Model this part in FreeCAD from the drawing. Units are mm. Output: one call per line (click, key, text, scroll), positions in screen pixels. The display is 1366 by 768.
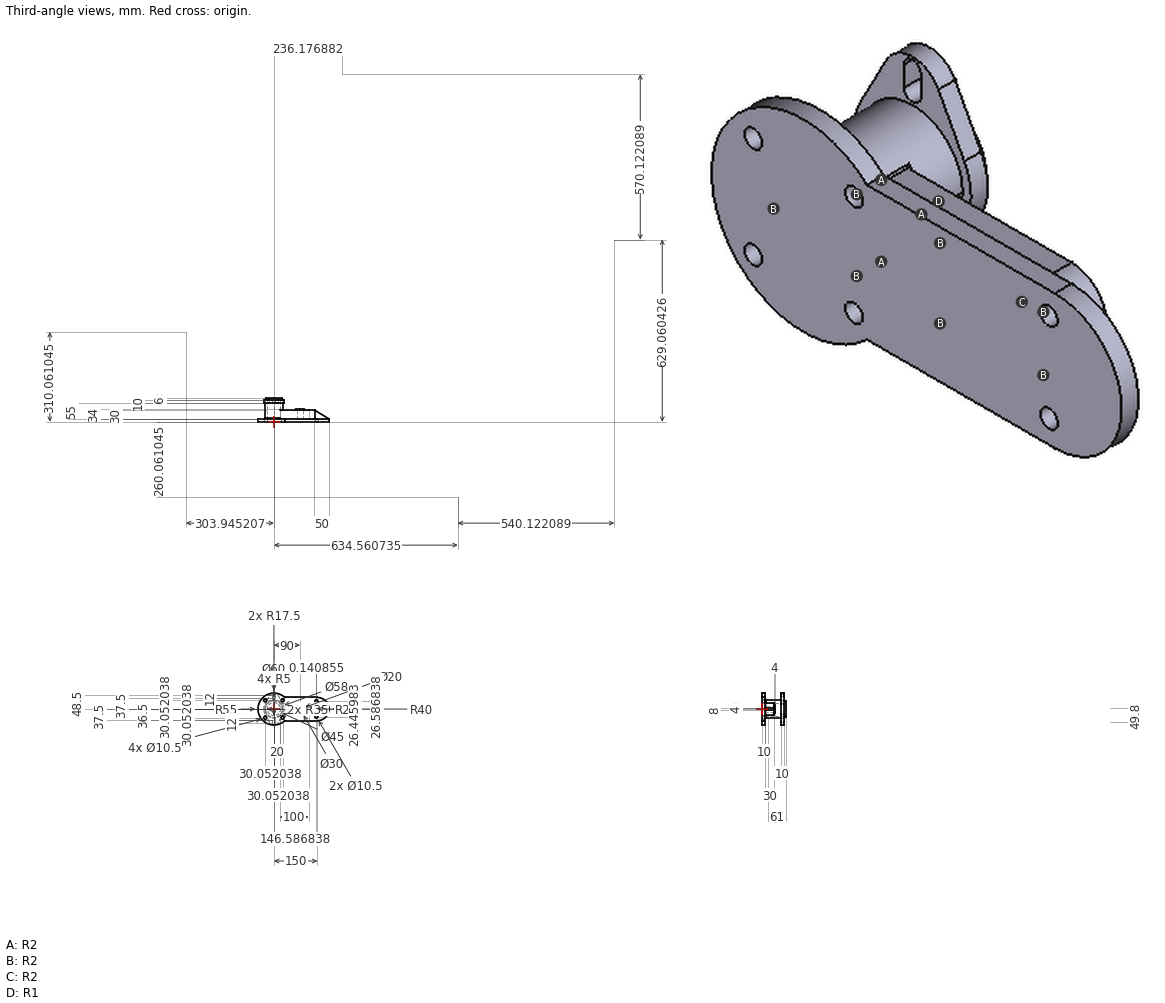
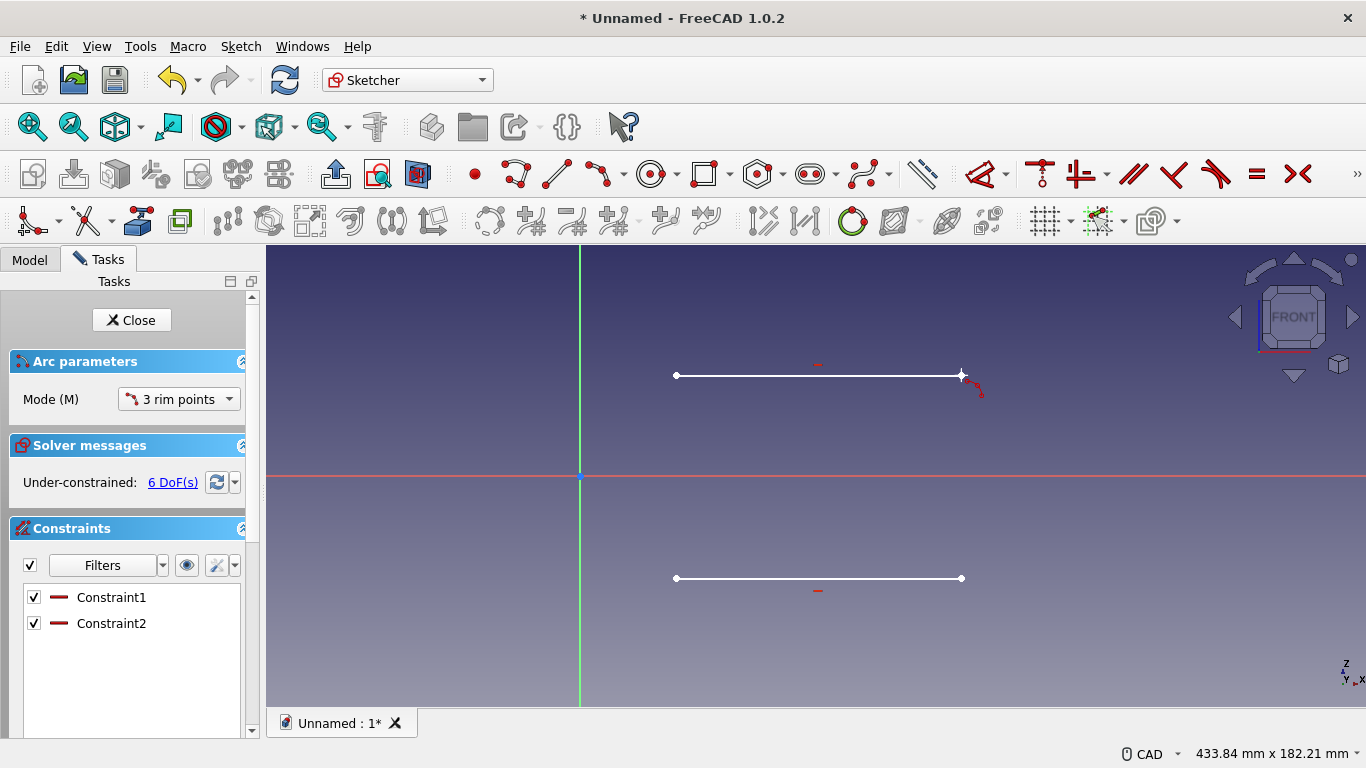
click(676, 579)
click(676, 376)
click(456, 414)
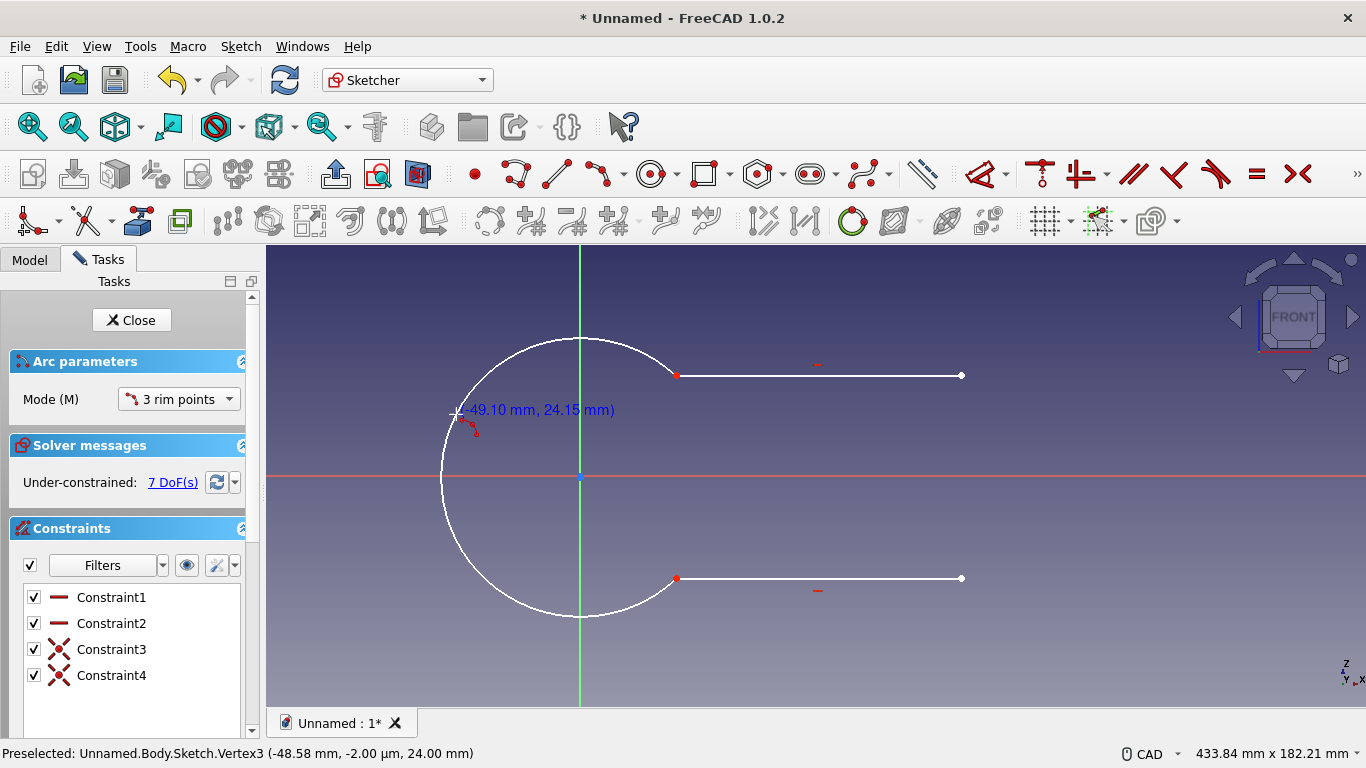
click(961, 376)
click(961, 579)
click(1057, 508)
key(Escape)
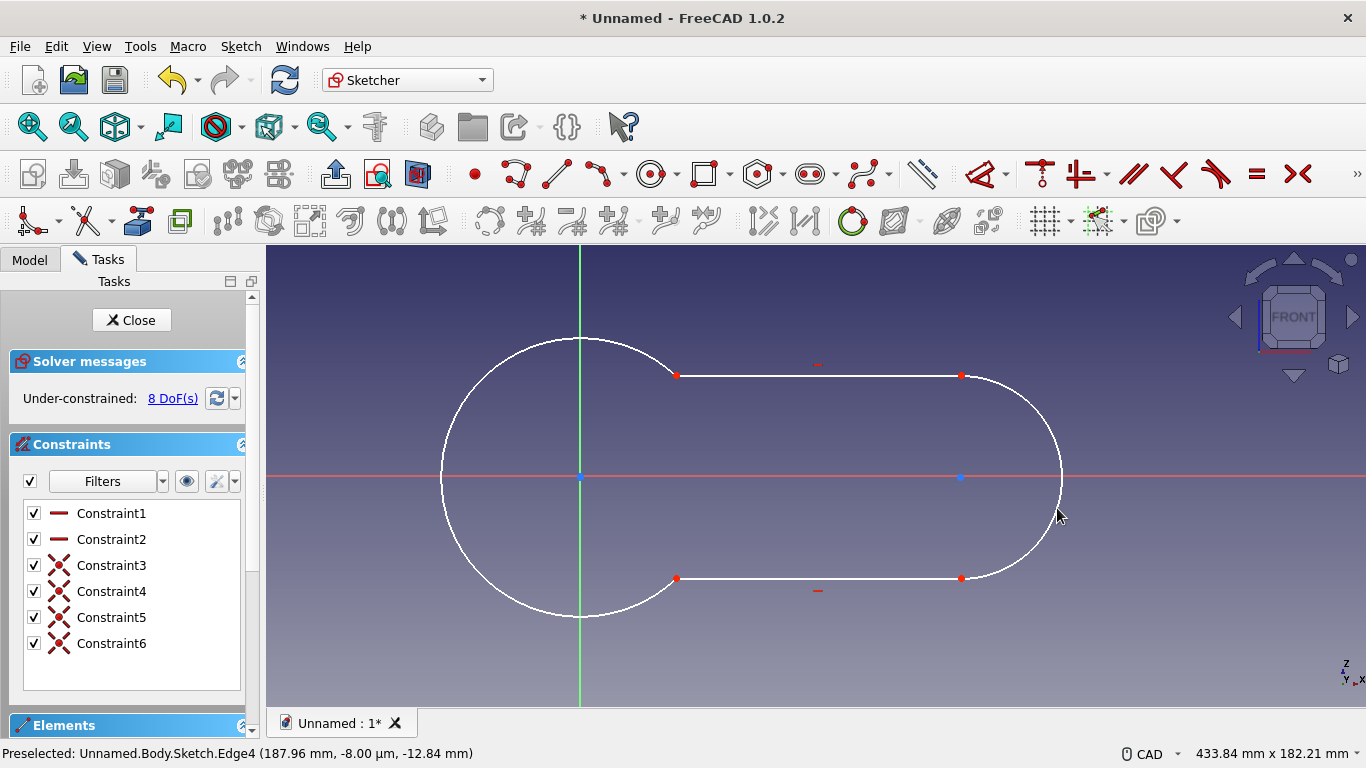
drag(570, 466, 591, 488)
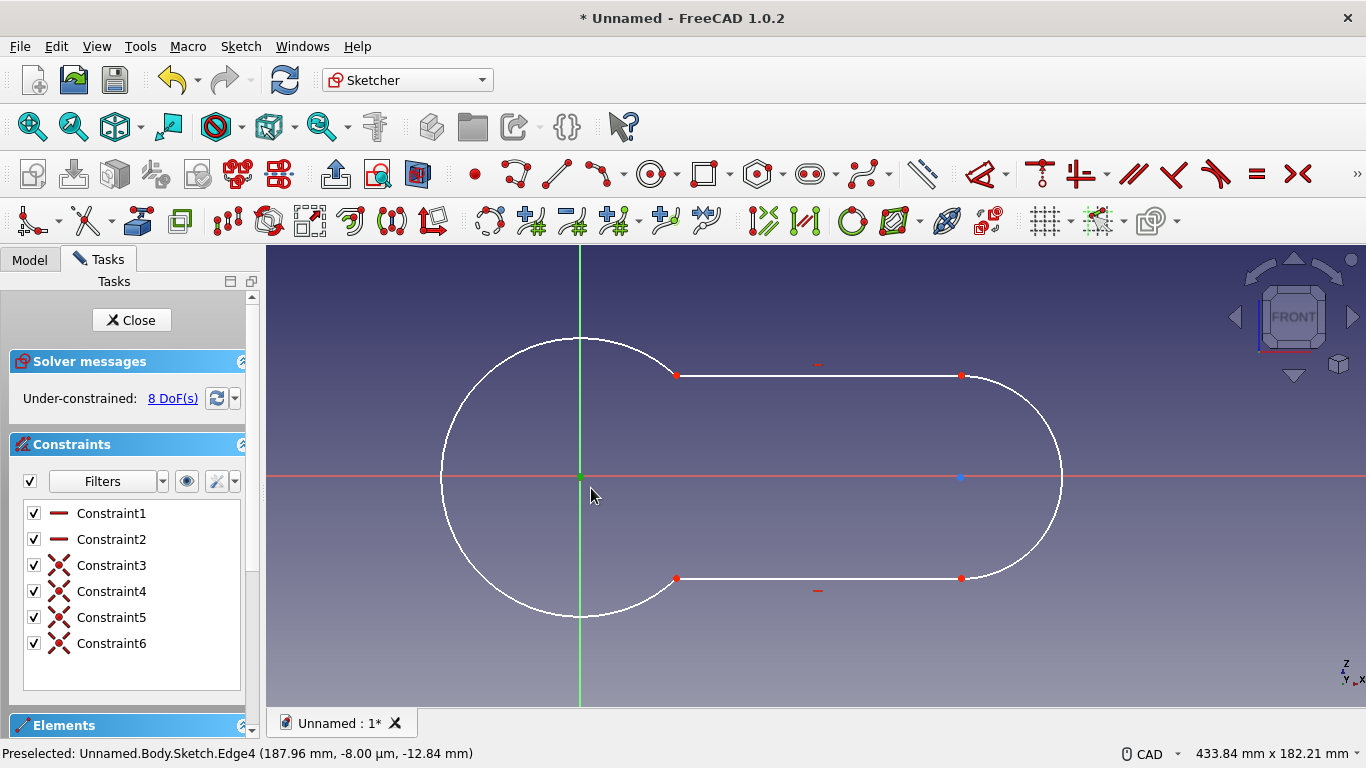
key(c)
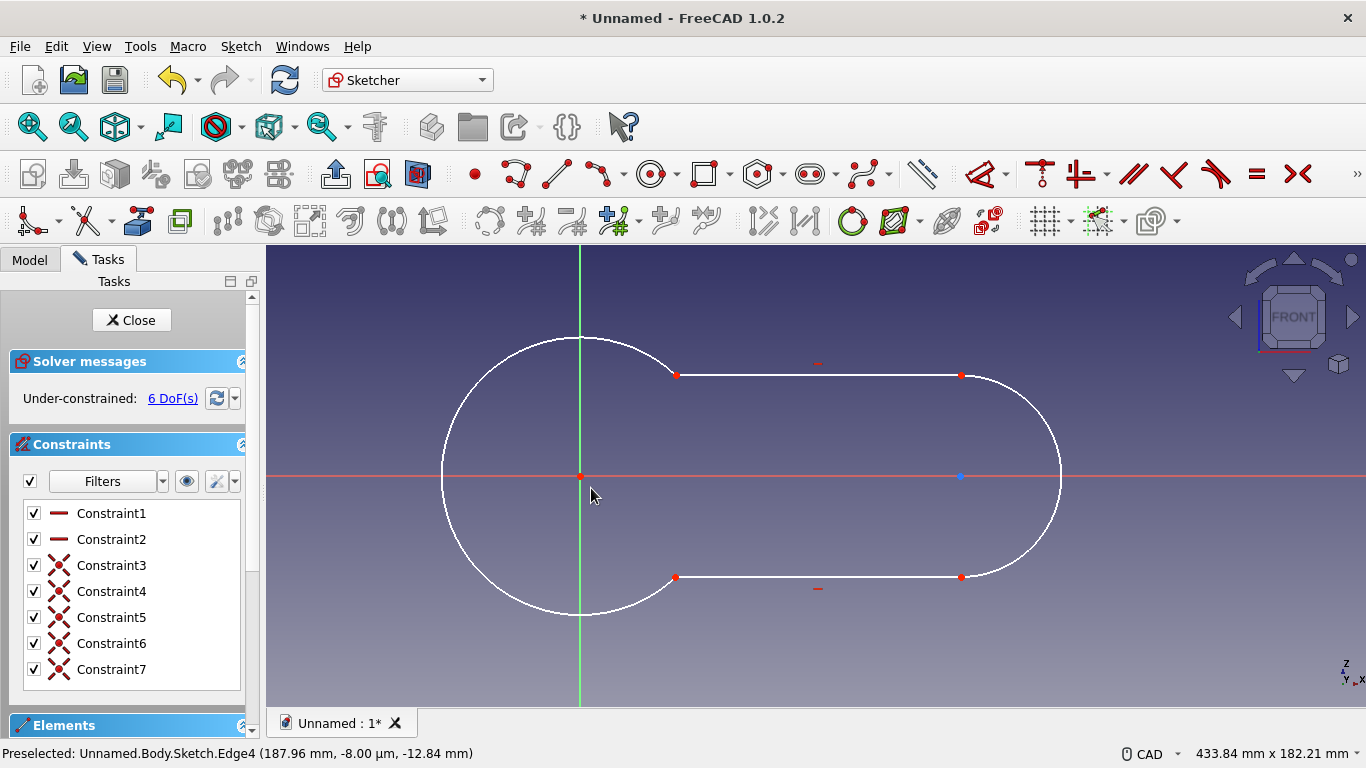
click(961, 476)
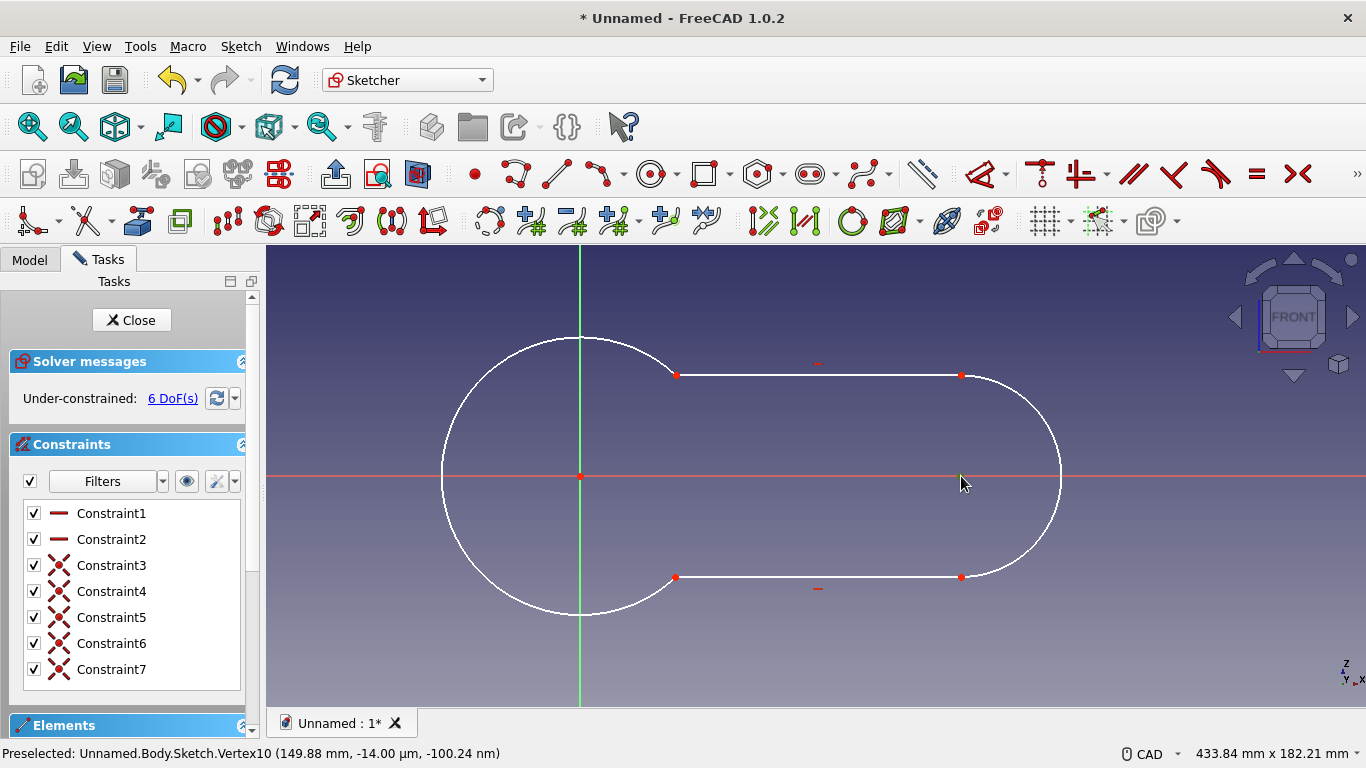
click(359, 476)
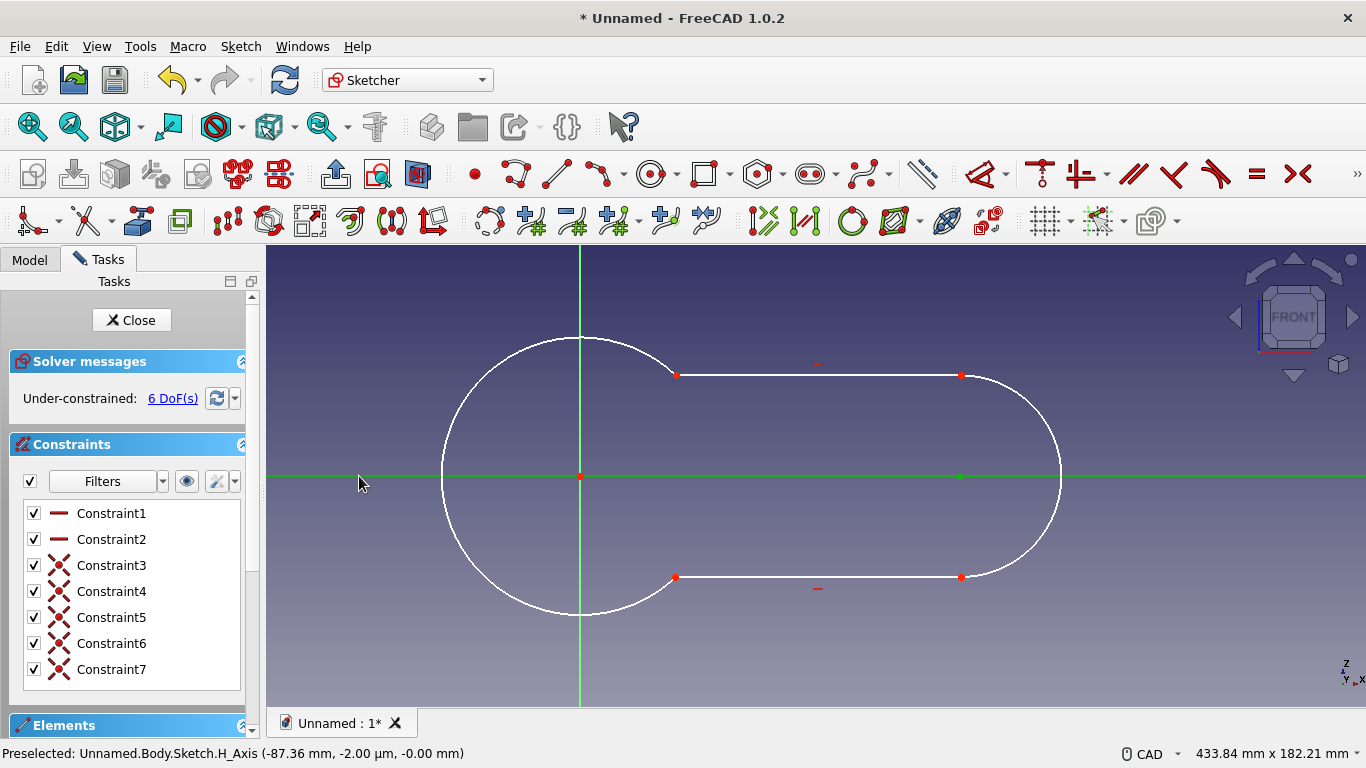
key(c)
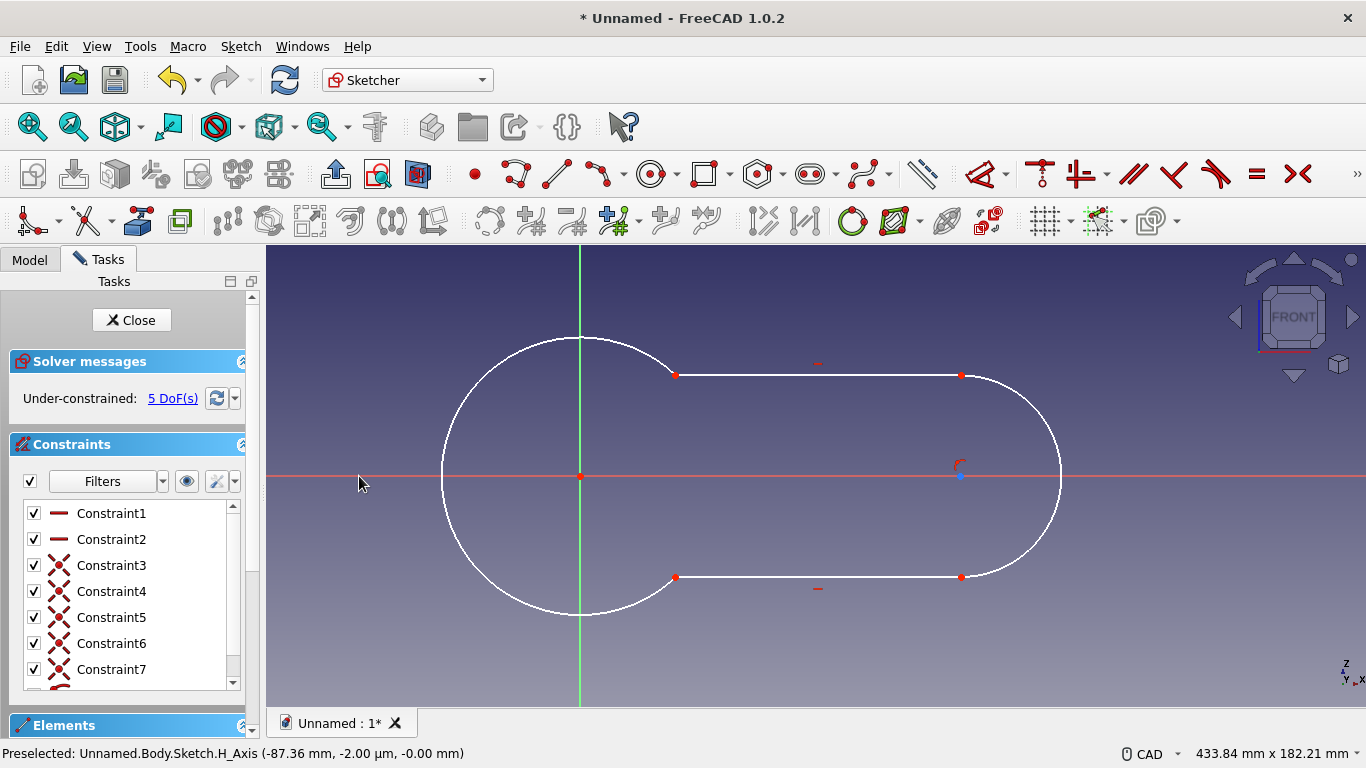
key(d)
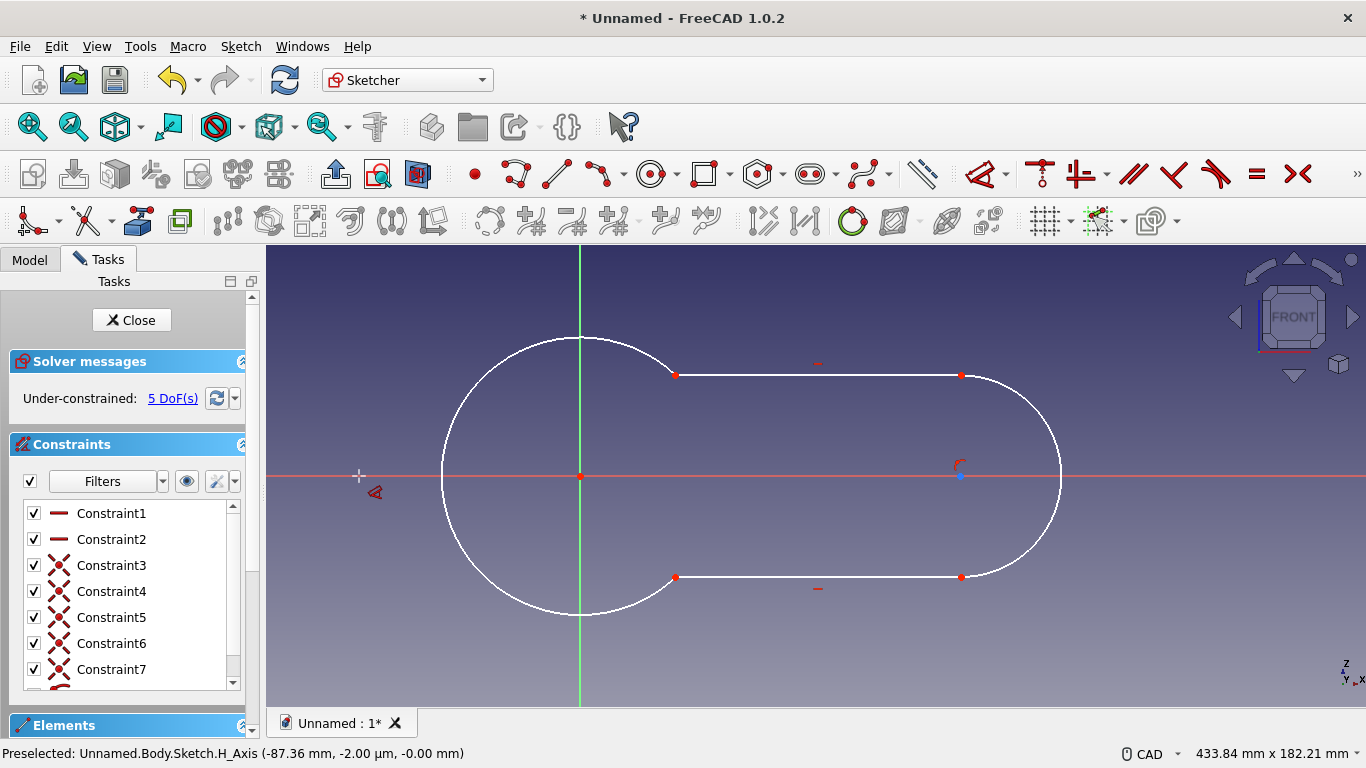
click(498, 365)
click(479, 339)